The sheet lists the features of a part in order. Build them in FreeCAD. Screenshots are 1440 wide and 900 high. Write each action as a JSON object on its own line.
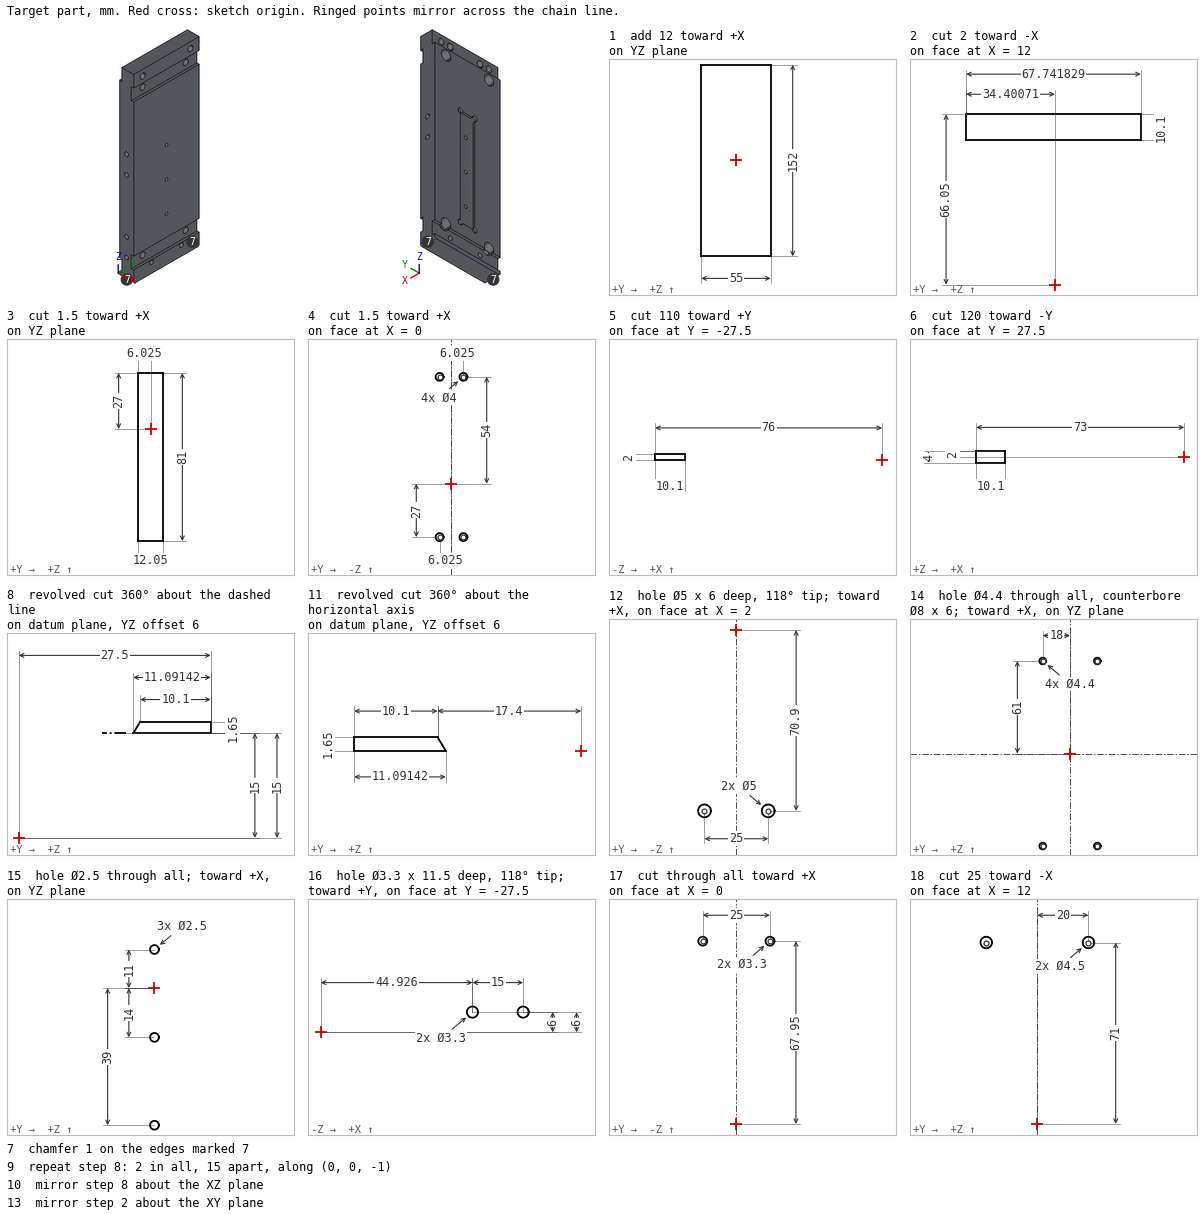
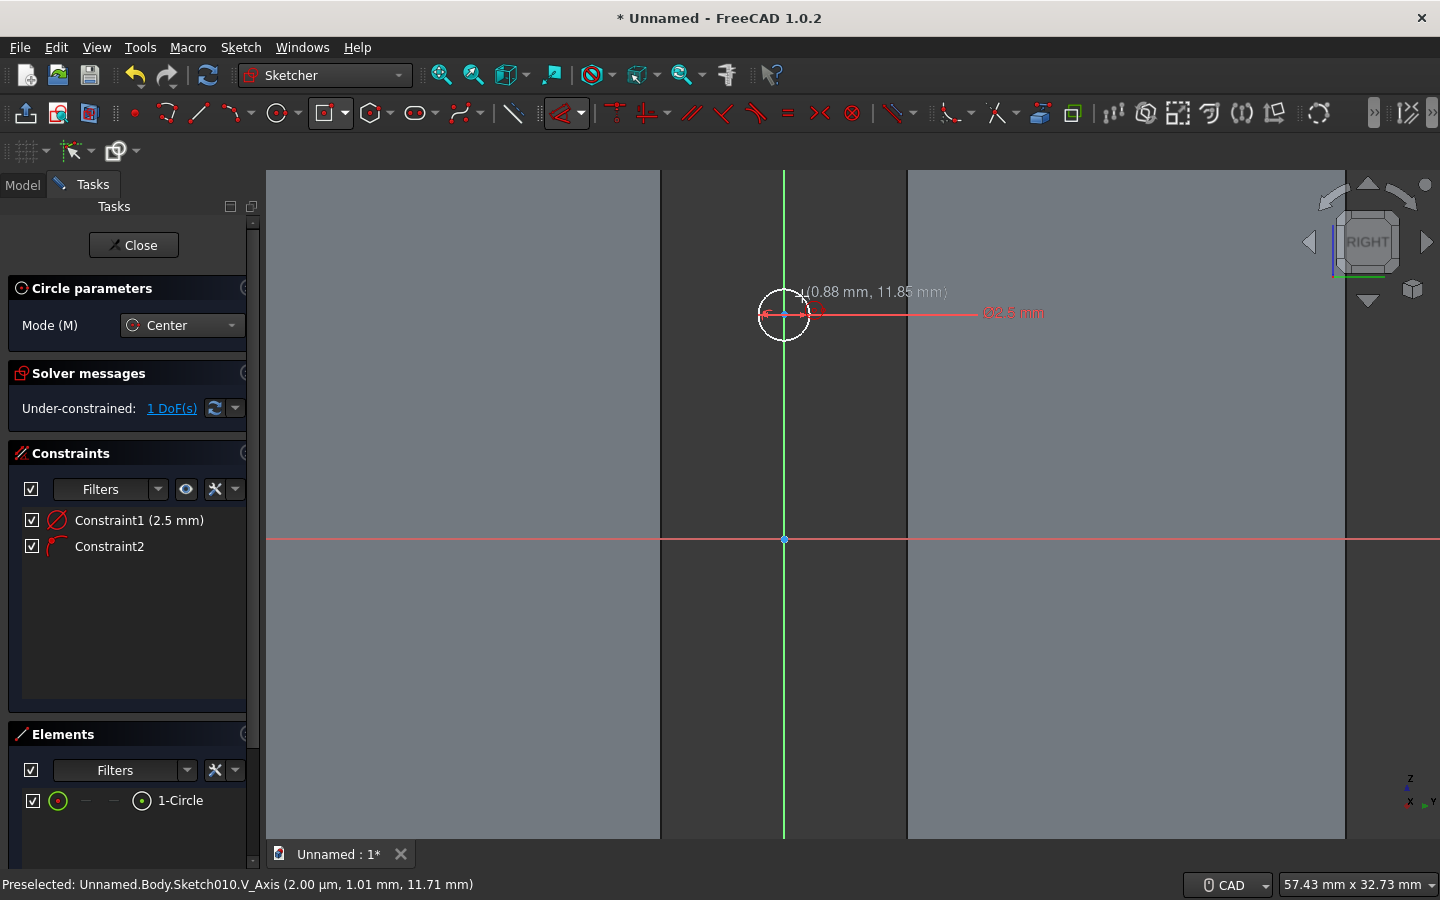
{"action": "scroll", "coordinate": [785, 318], "scroll_direction": "down", "scroll_amount": 5}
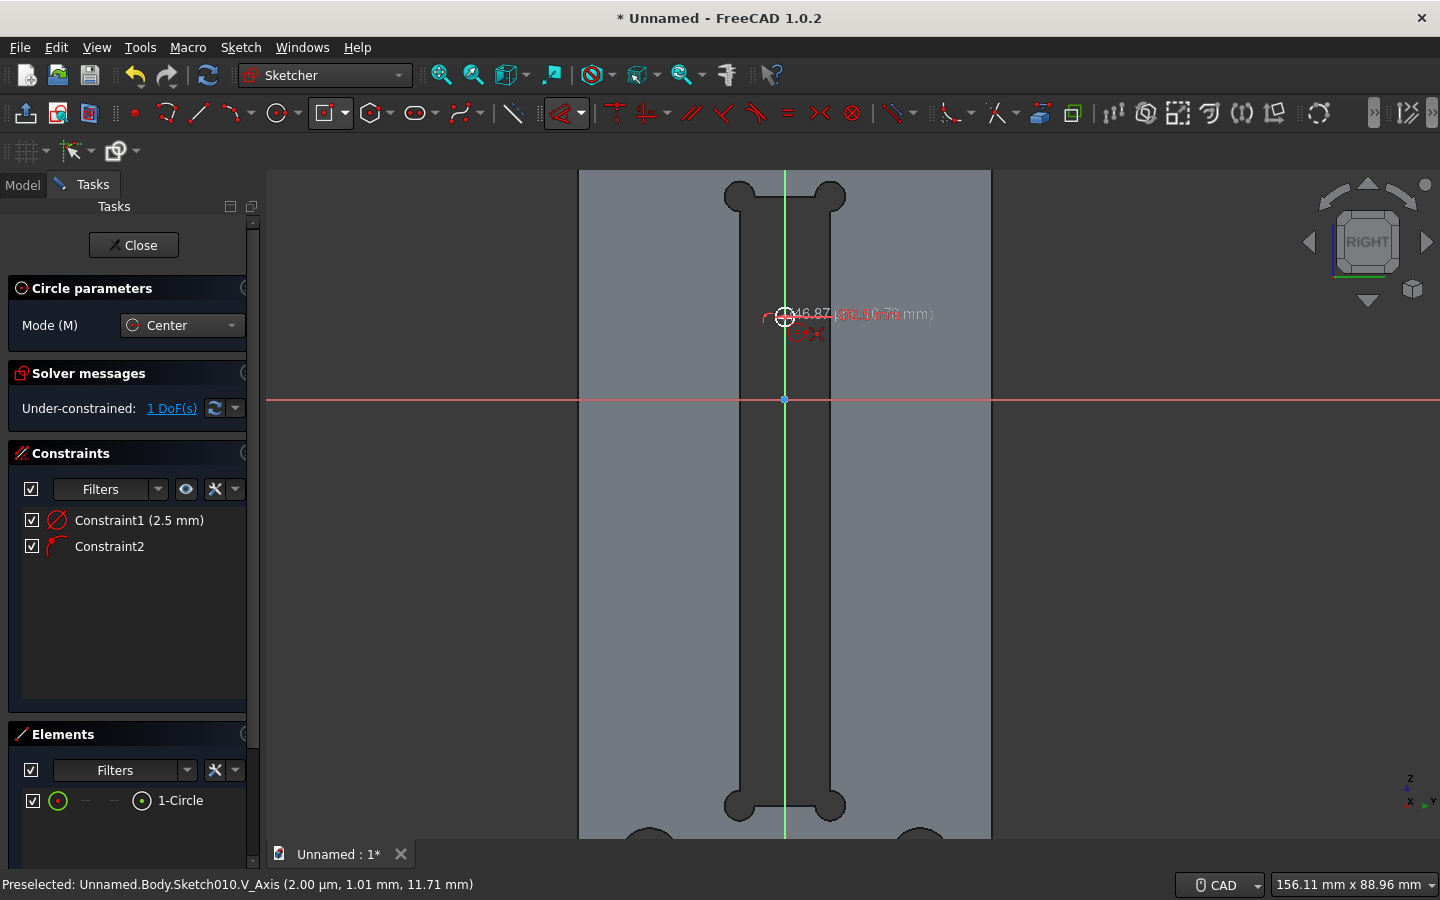
{"action": "scroll", "coordinate": [785, 505], "scroll_direction": "up", "scroll_amount": 5}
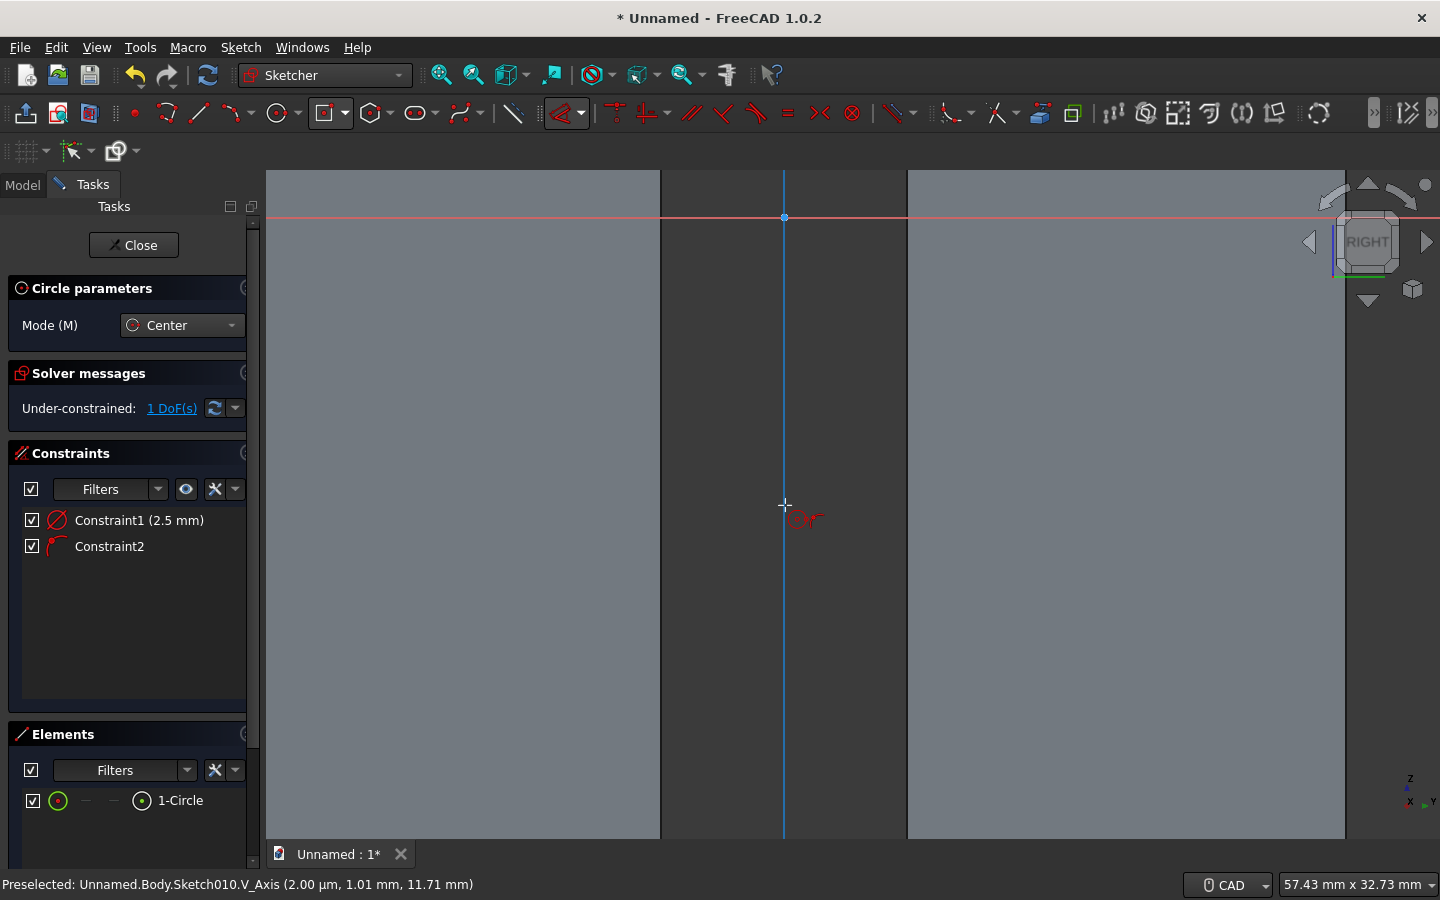
{"action": "left_click", "coordinate": [784, 504]}
{"action": "mouse_move", "coordinate": [802, 486]}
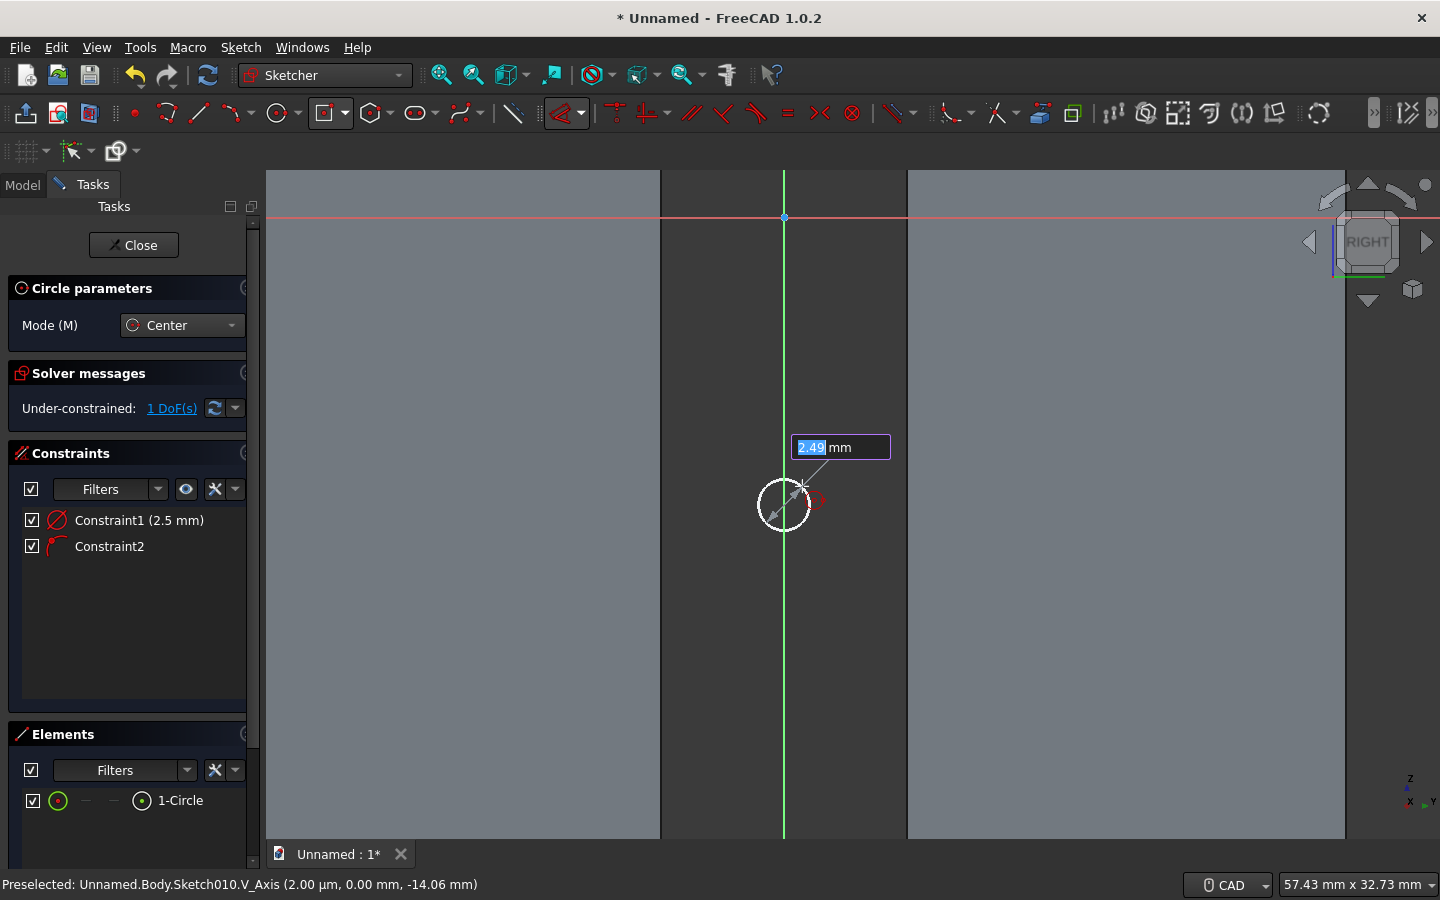
{"action": "type", "text": "2.5"}
{"action": "key", "text": "Return"}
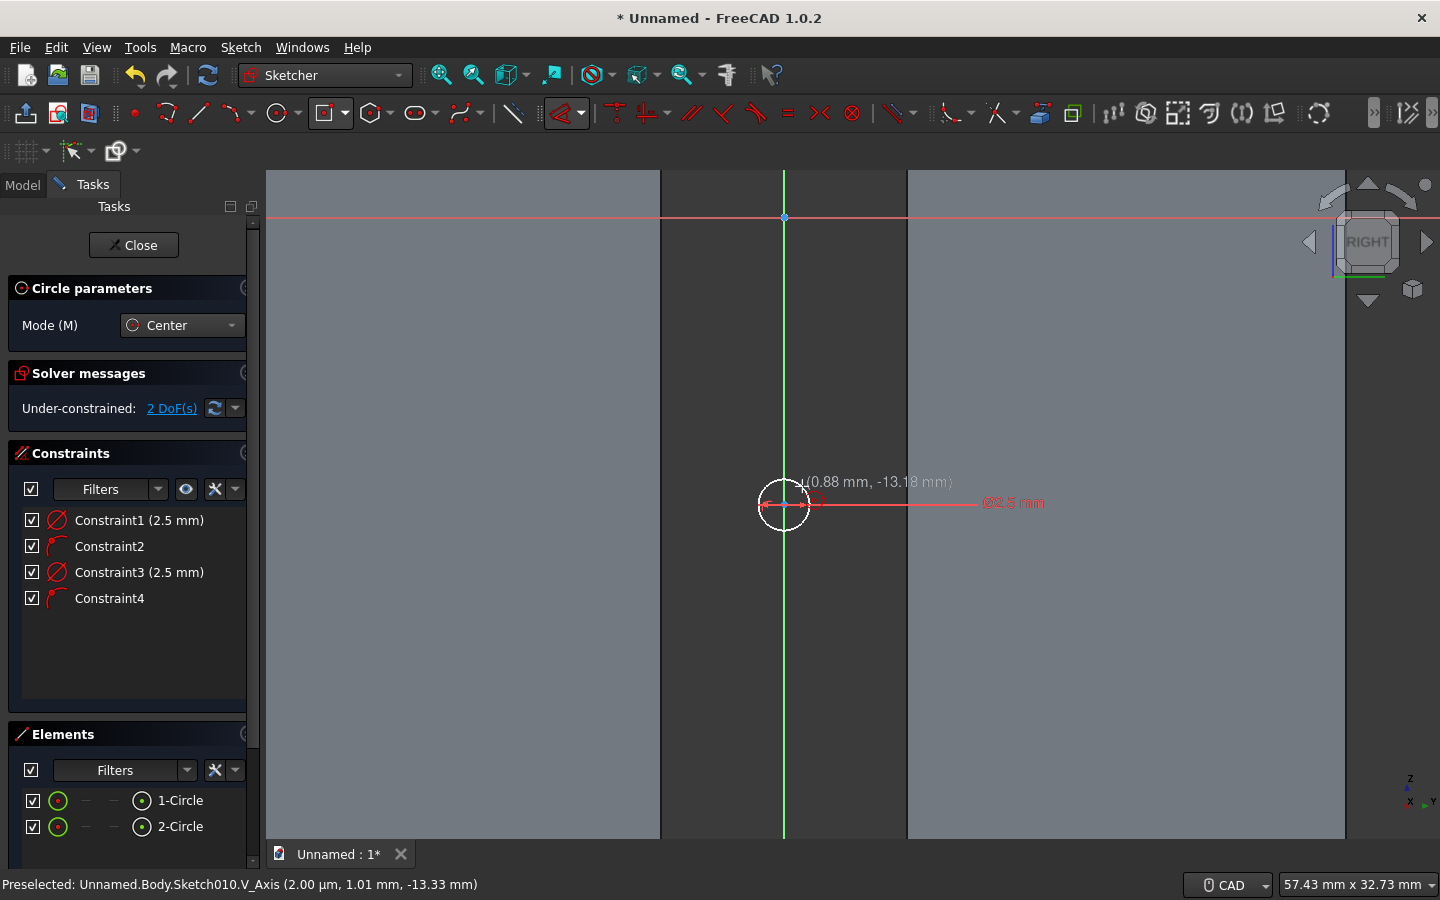
{"action": "scroll", "coordinate": [785, 505], "scroll_direction": "down", "scroll_amount": 5}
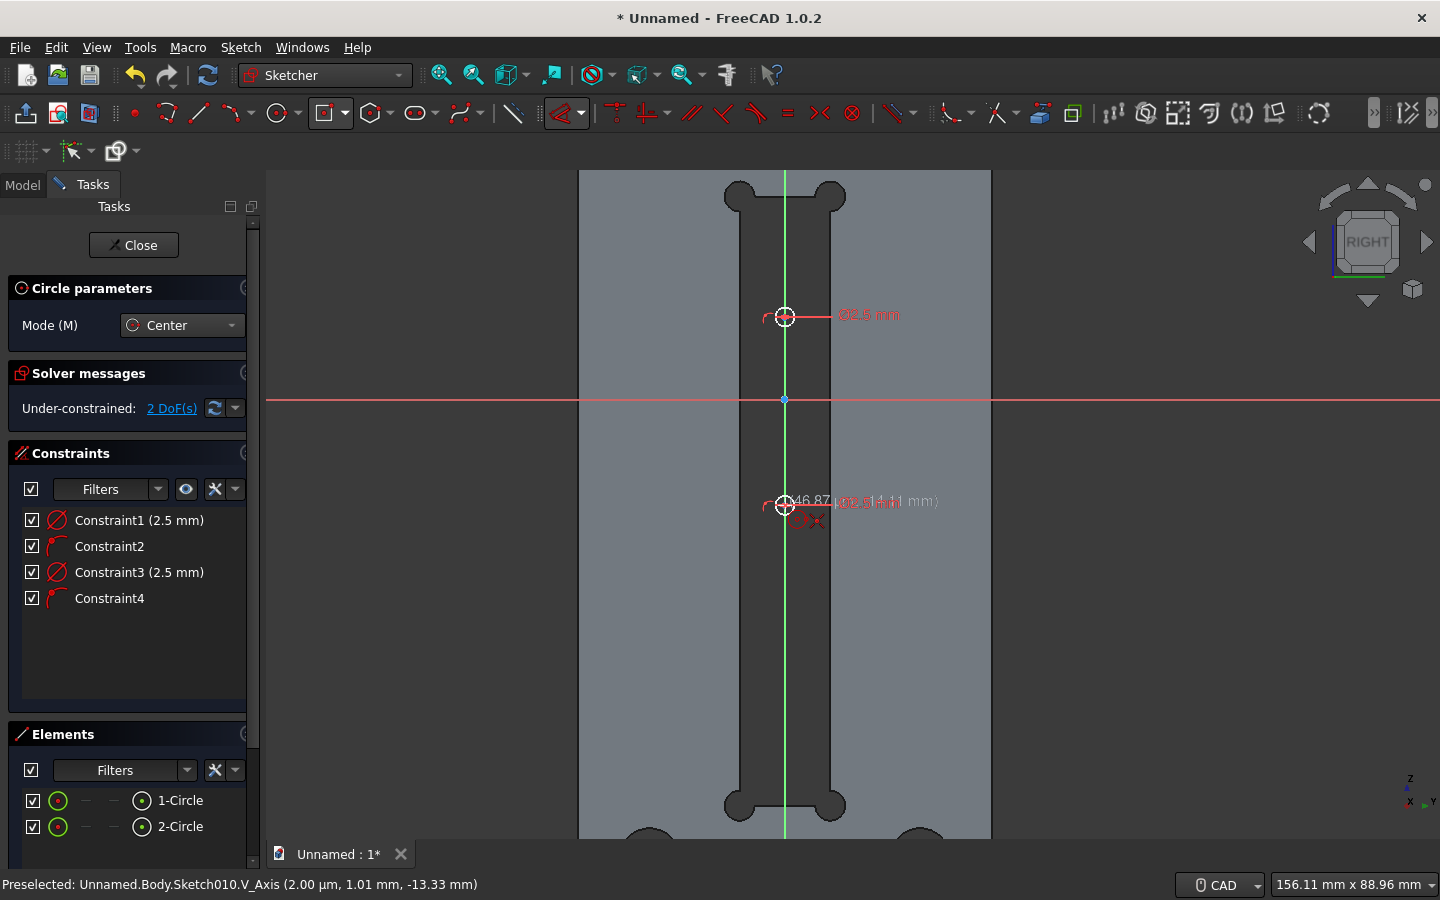
{"action": "scroll", "coordinate": [785, 693], "scroll_direction": "up", "scroll_amount": 5}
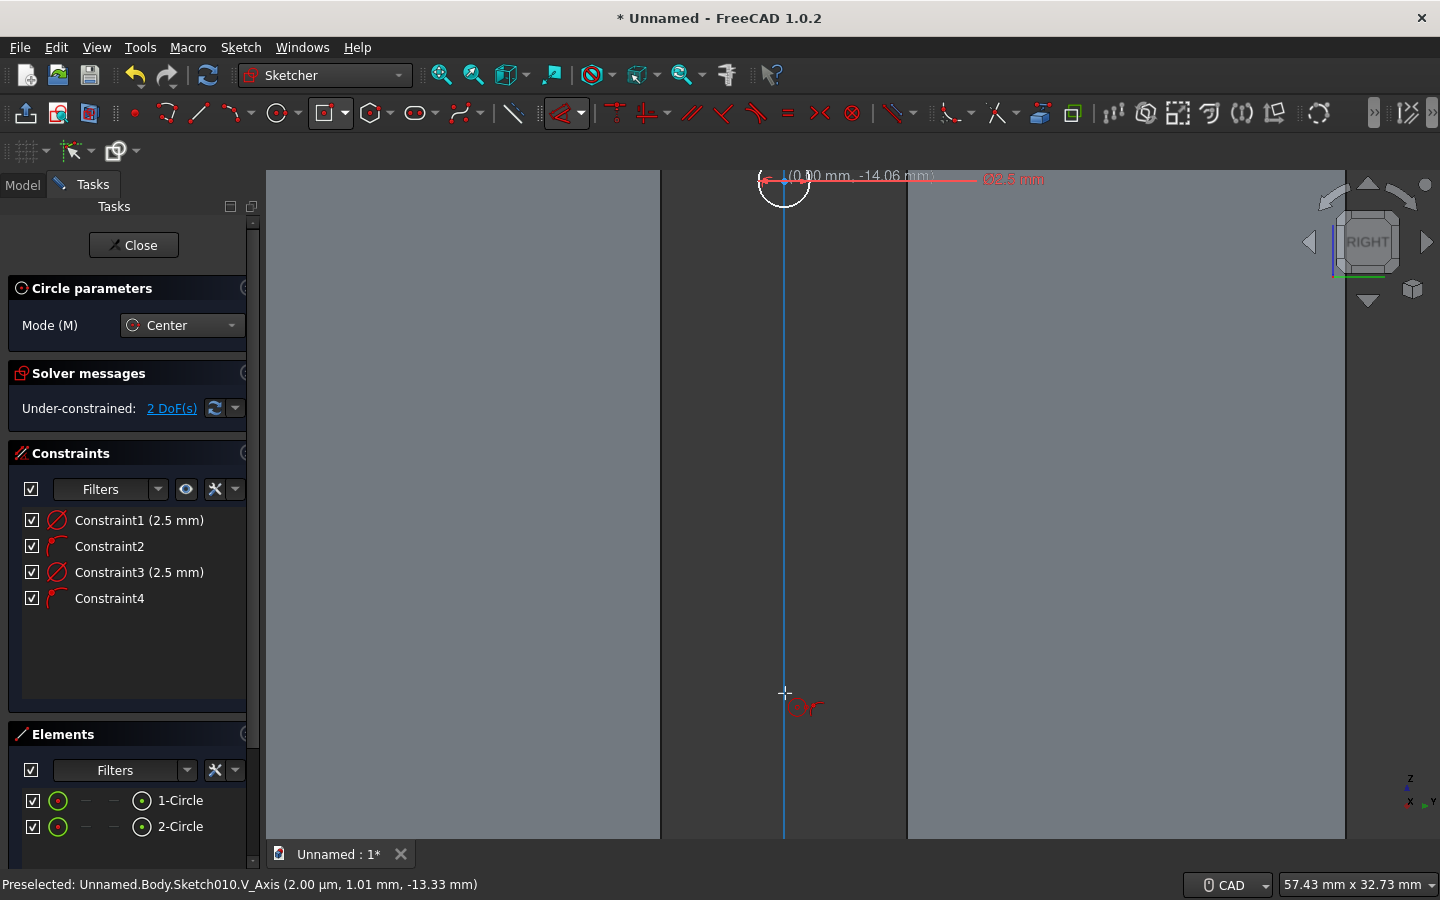
{"action": "left_click", "coordinate": [784, 691]}
{"action": "mouse_move", "coordinate": [802, 673]}